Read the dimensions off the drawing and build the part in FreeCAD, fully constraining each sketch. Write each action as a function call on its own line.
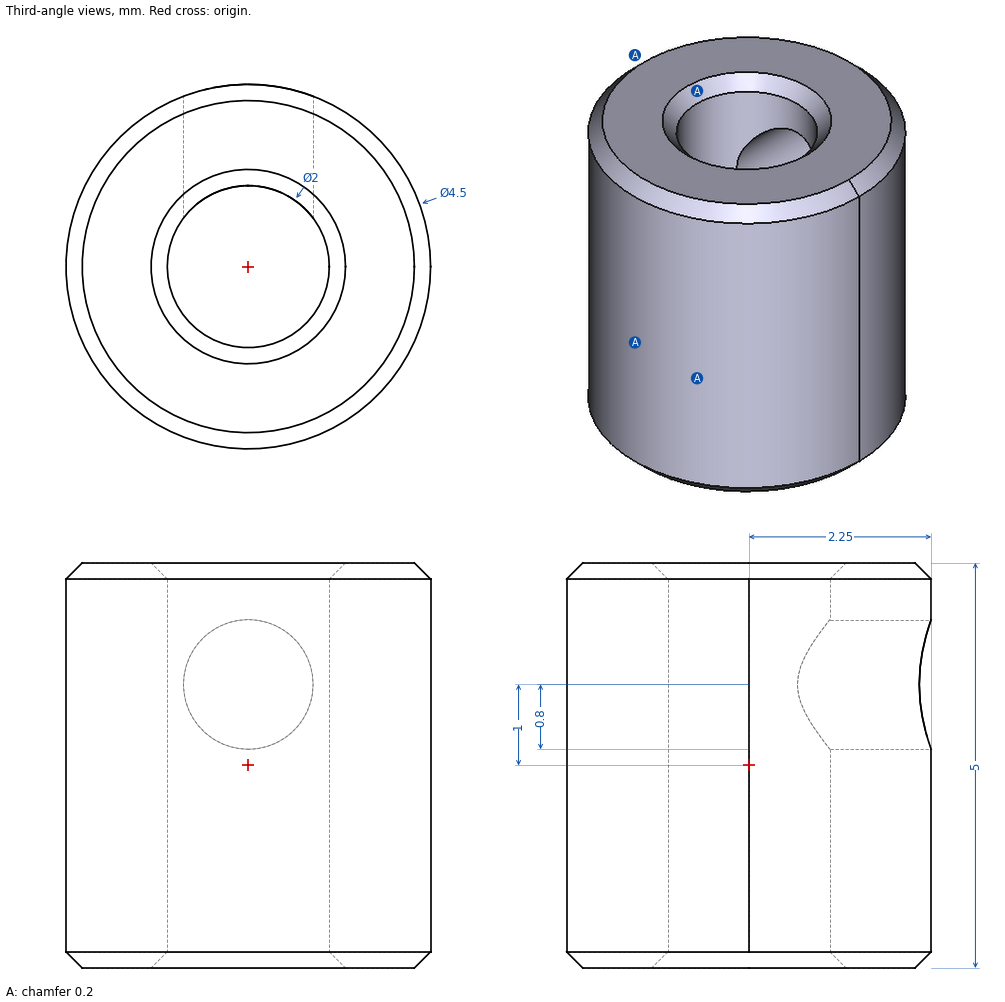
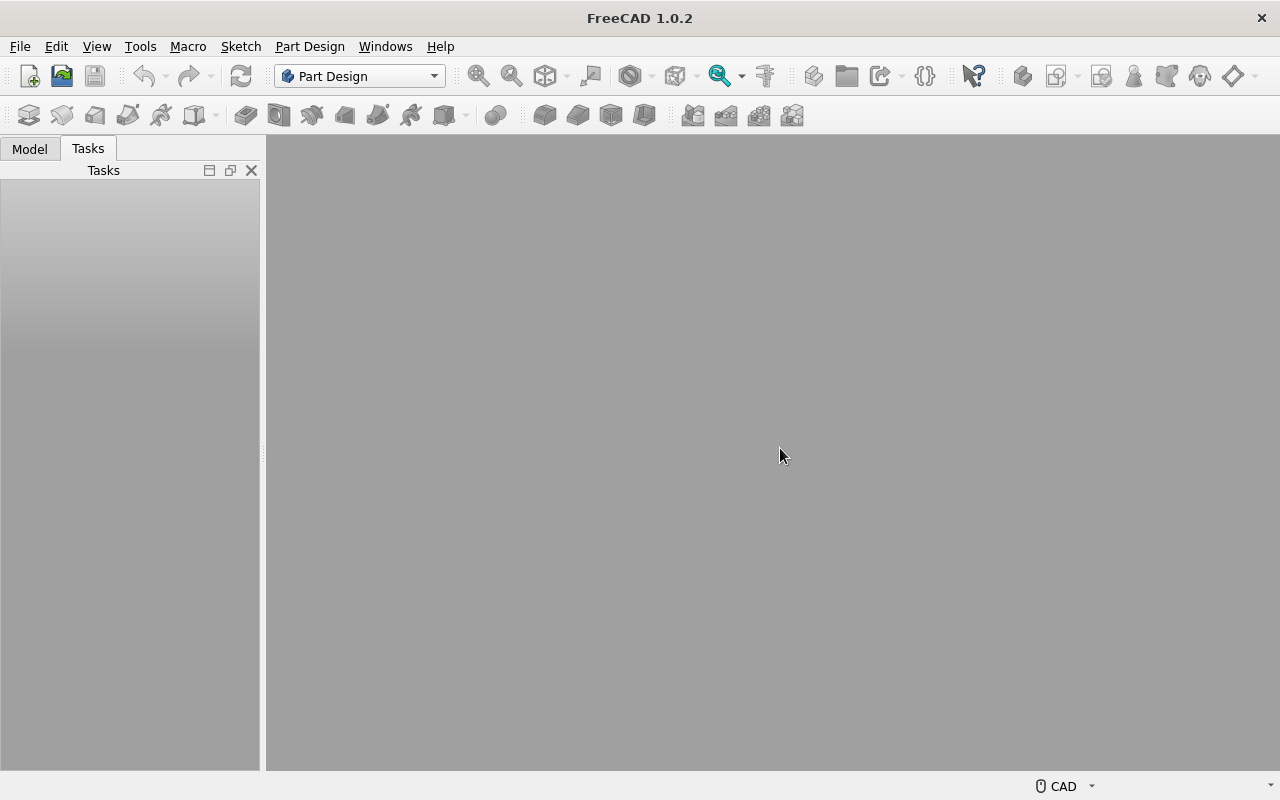
click(29, 76)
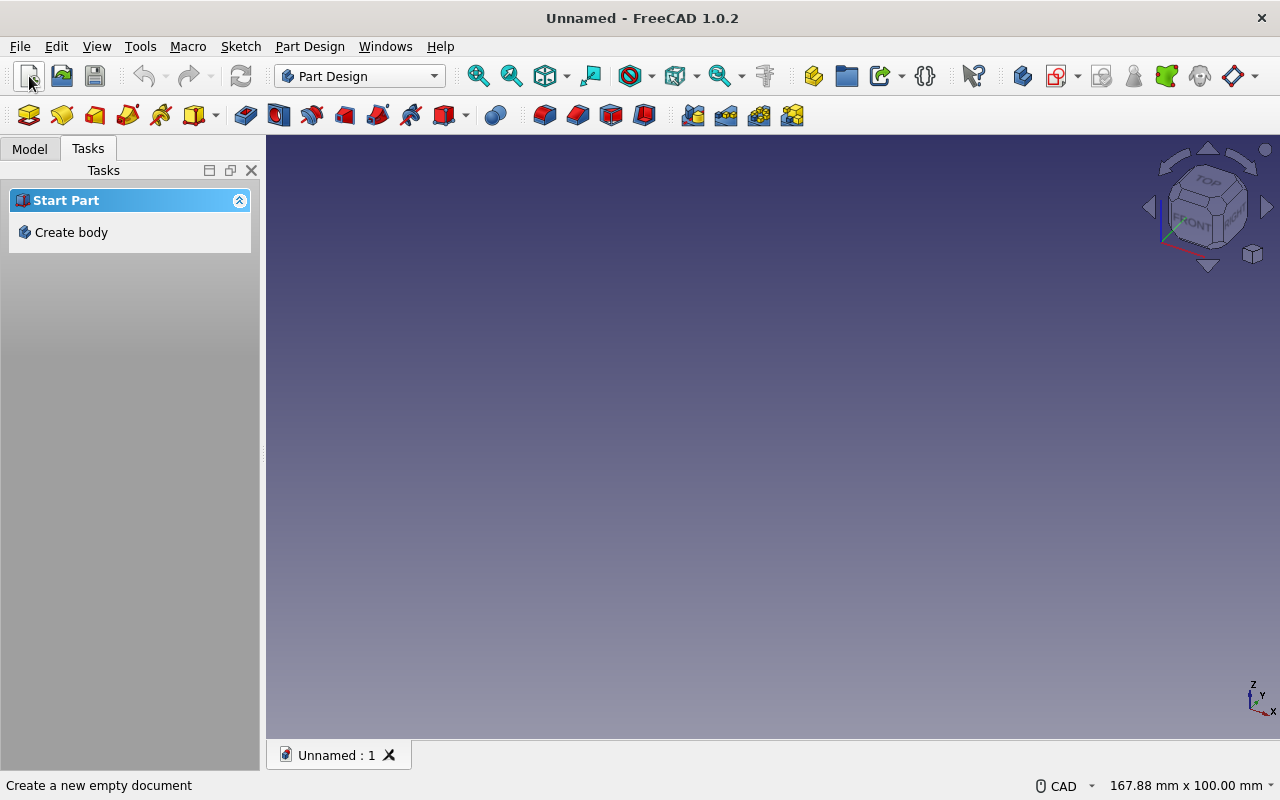
click(1056, 76)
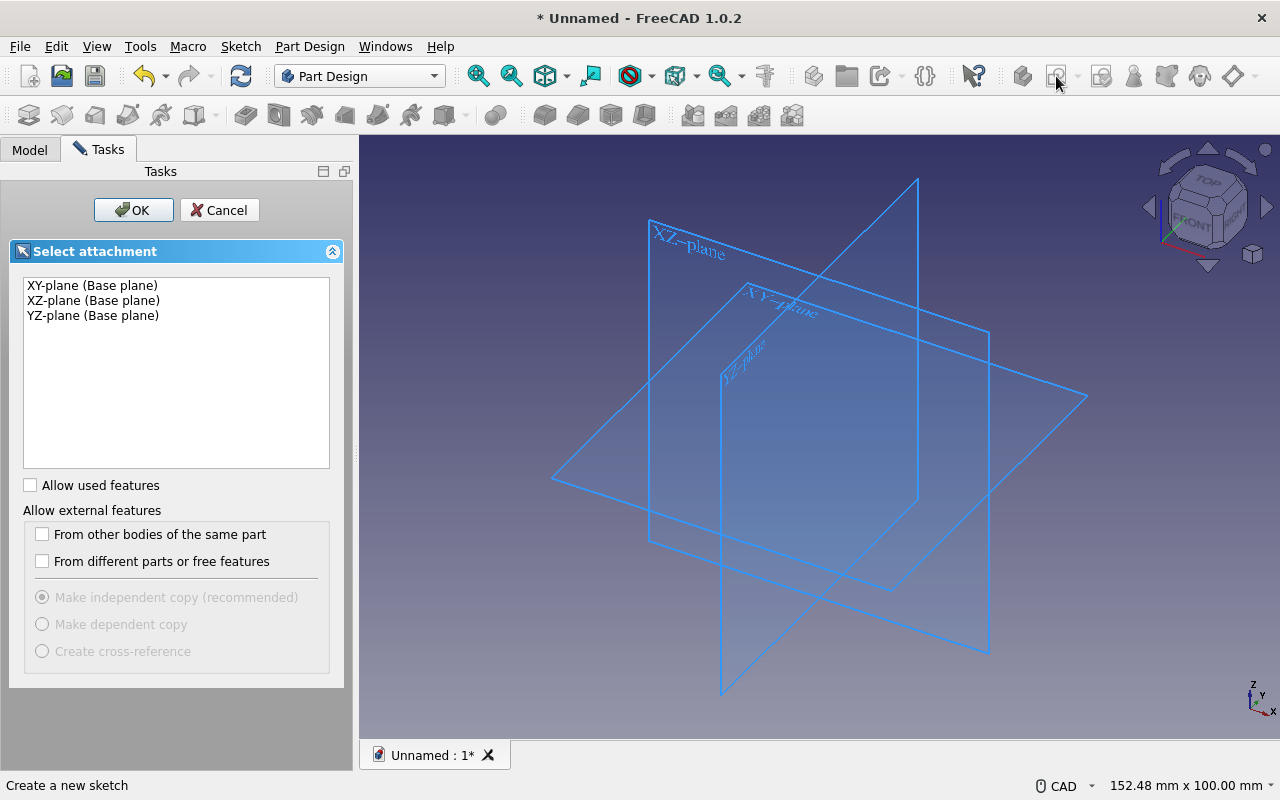
click(84, 286)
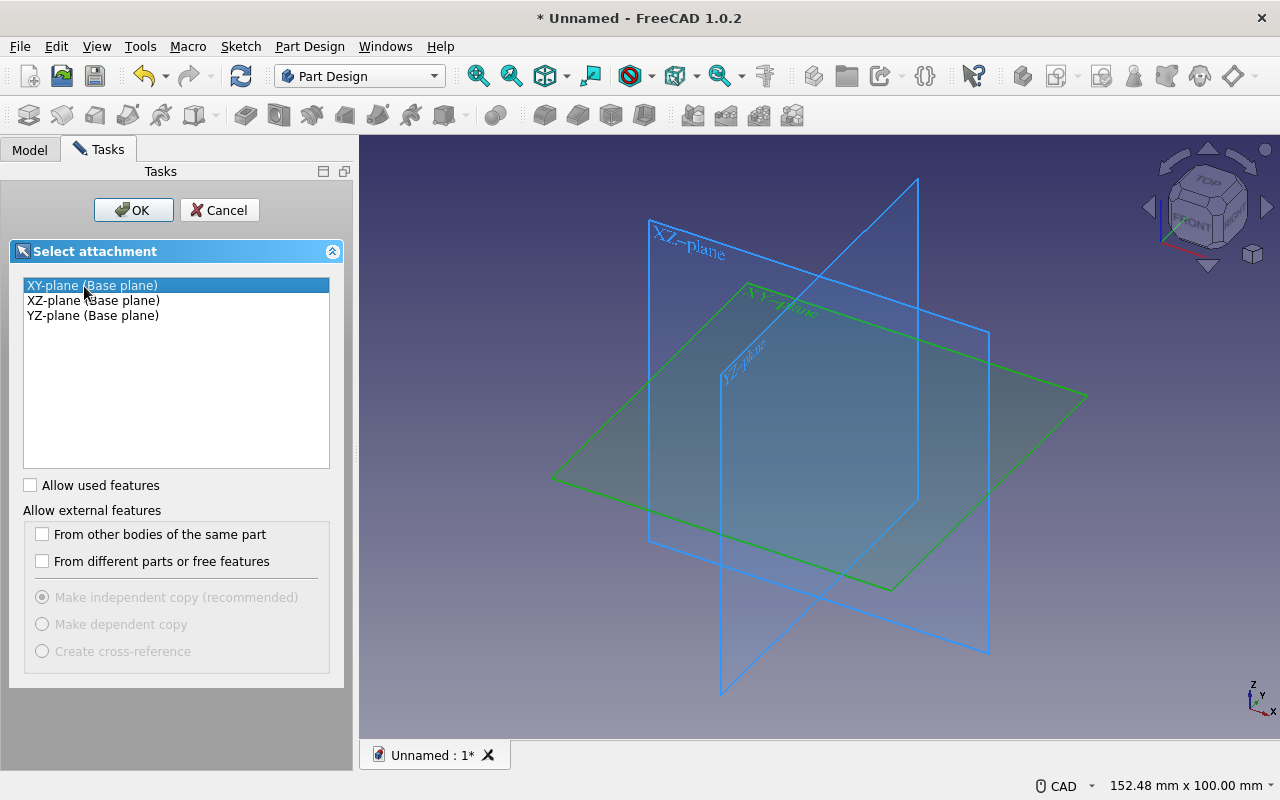
click(134, 210)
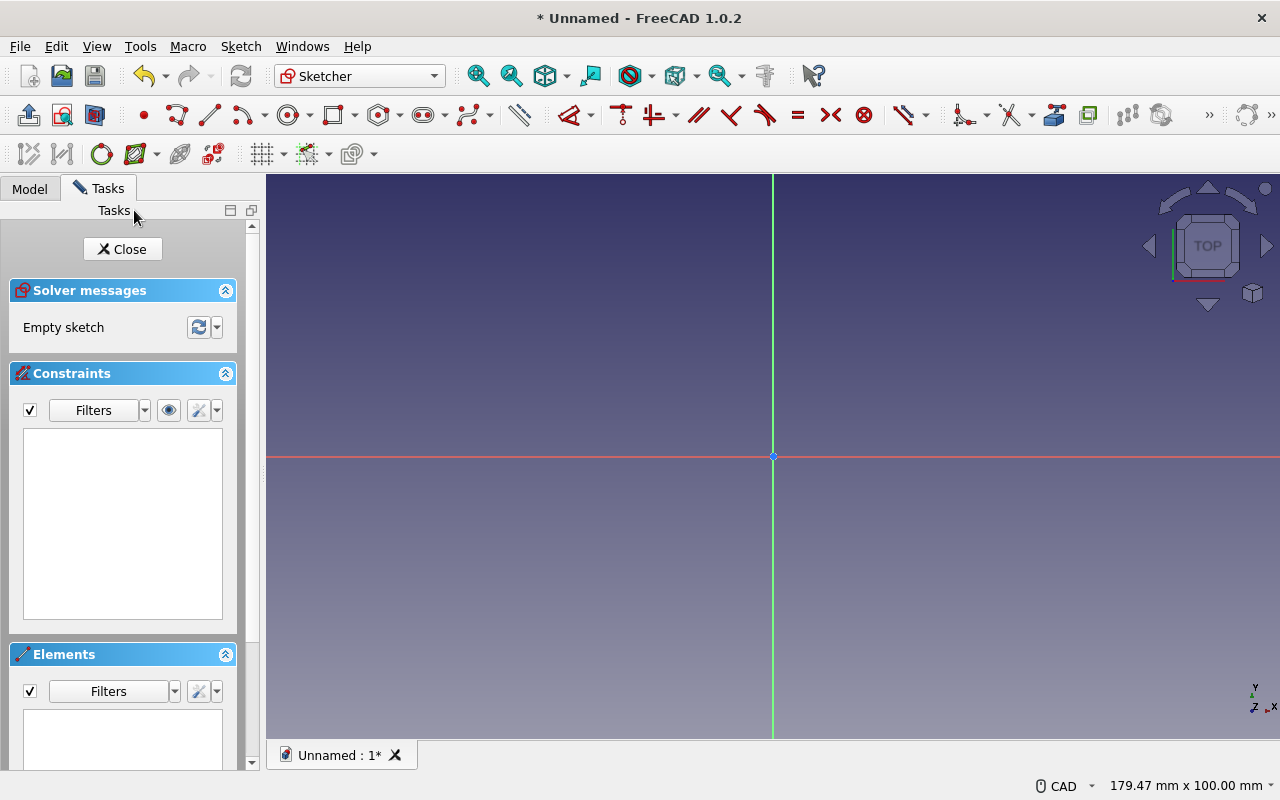
scroll(778, 456, up, 13)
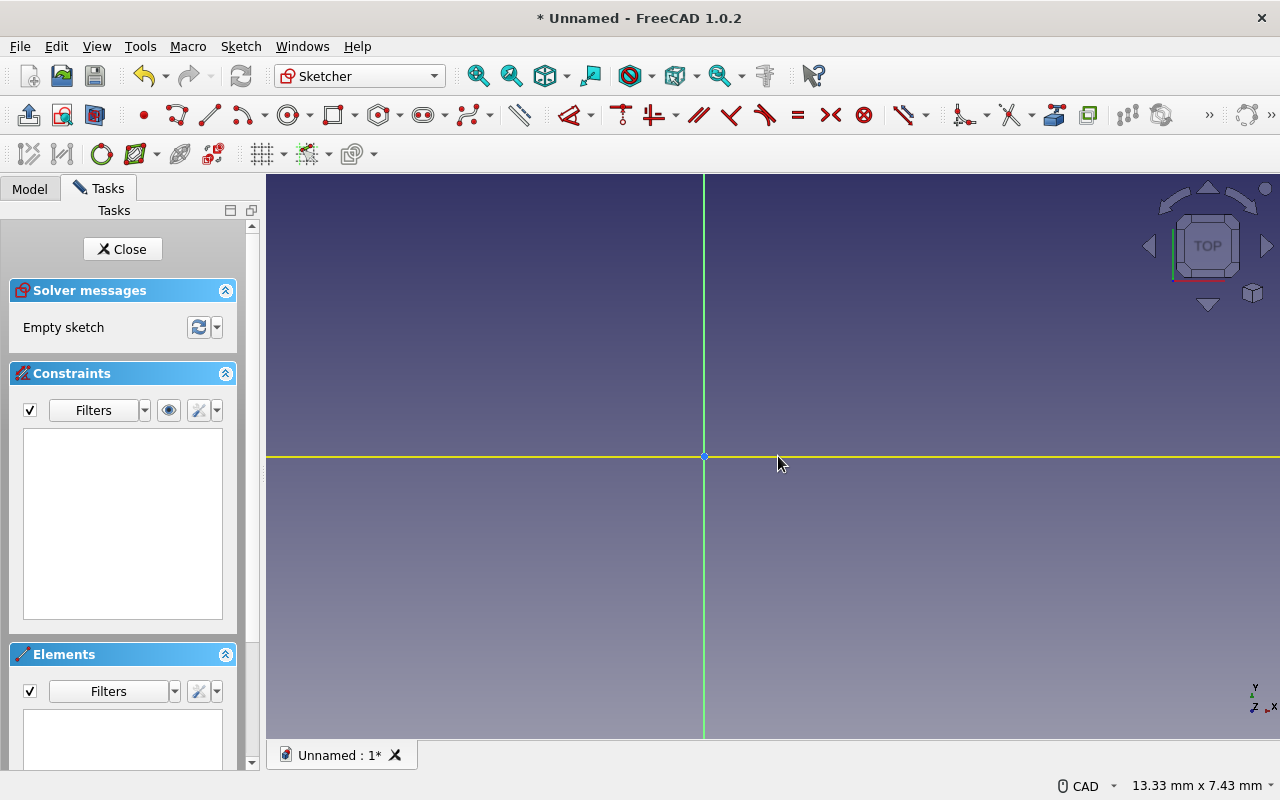
click(288, 116)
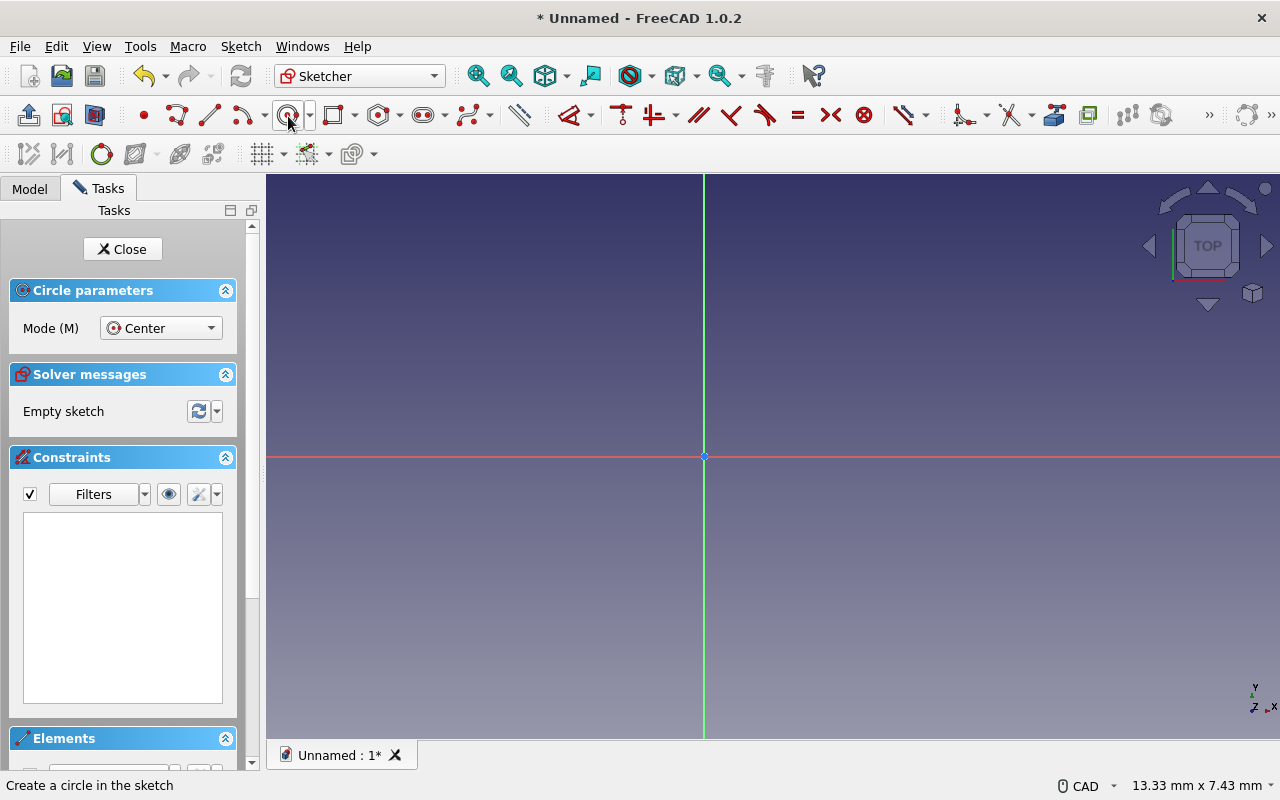
click(704, 456)
click(825, 335)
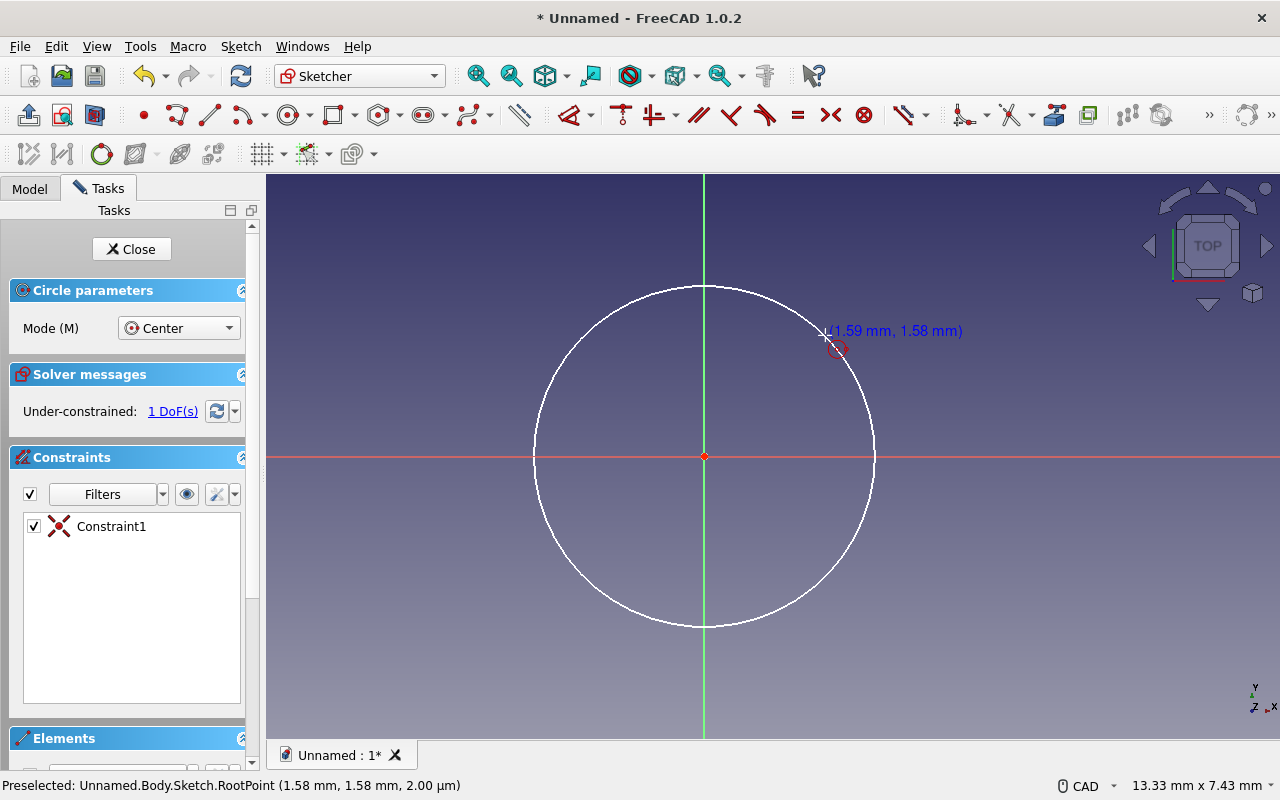
click(704, 456)
click(758, 403)
key(Escape)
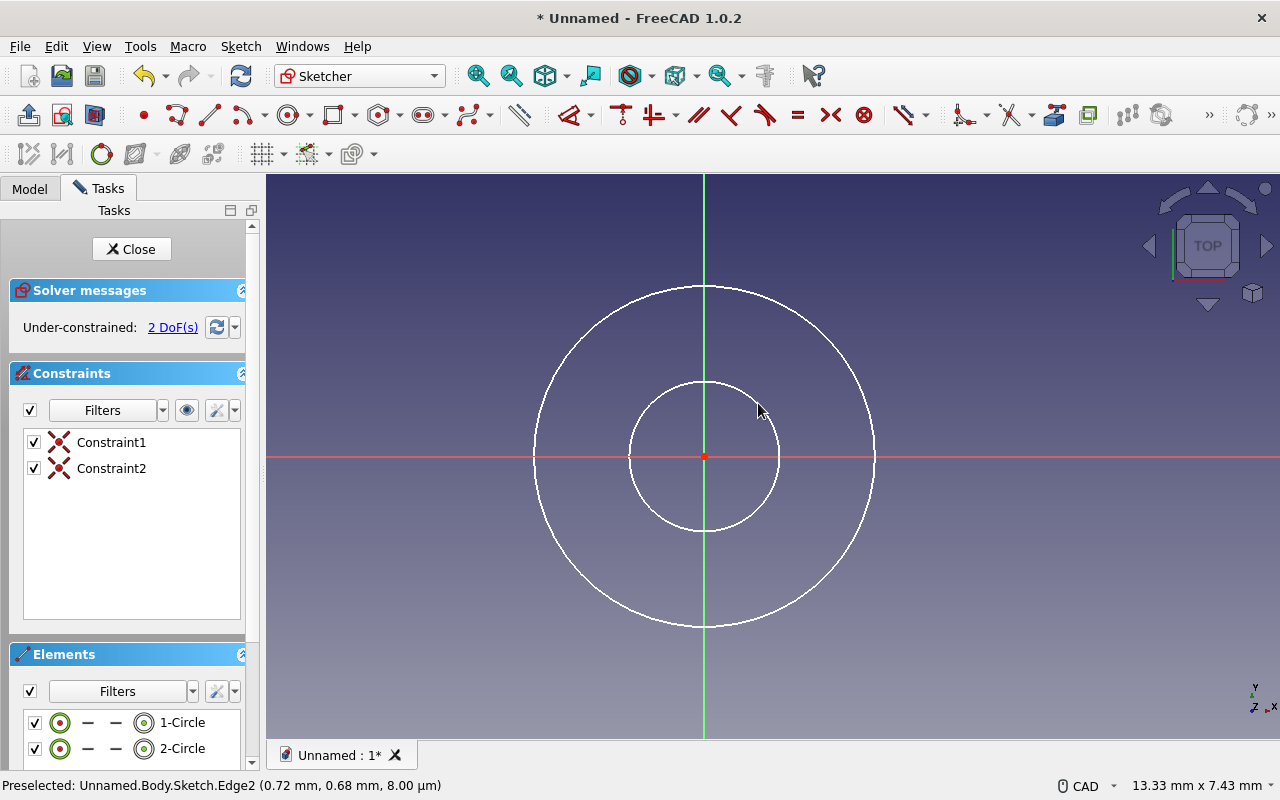
click(568, 116)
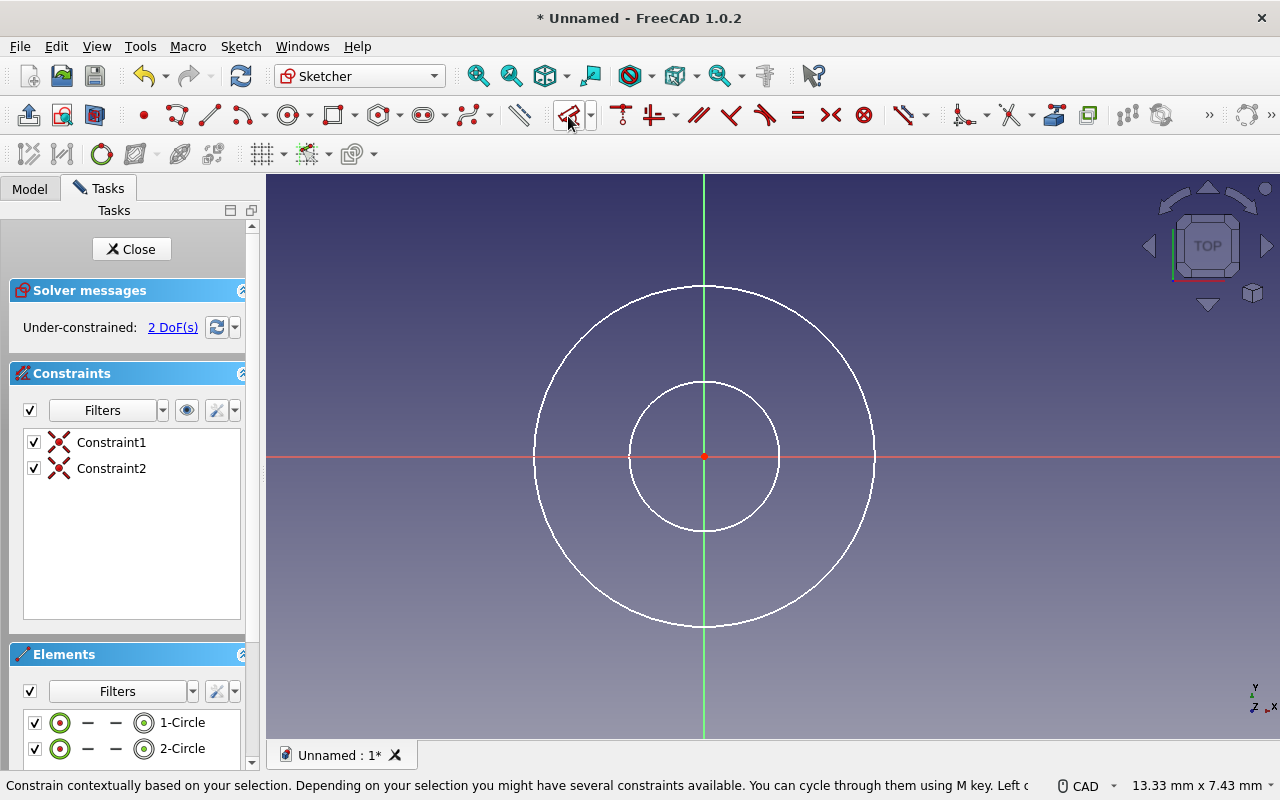
click(825, 336)
click(848, 313)